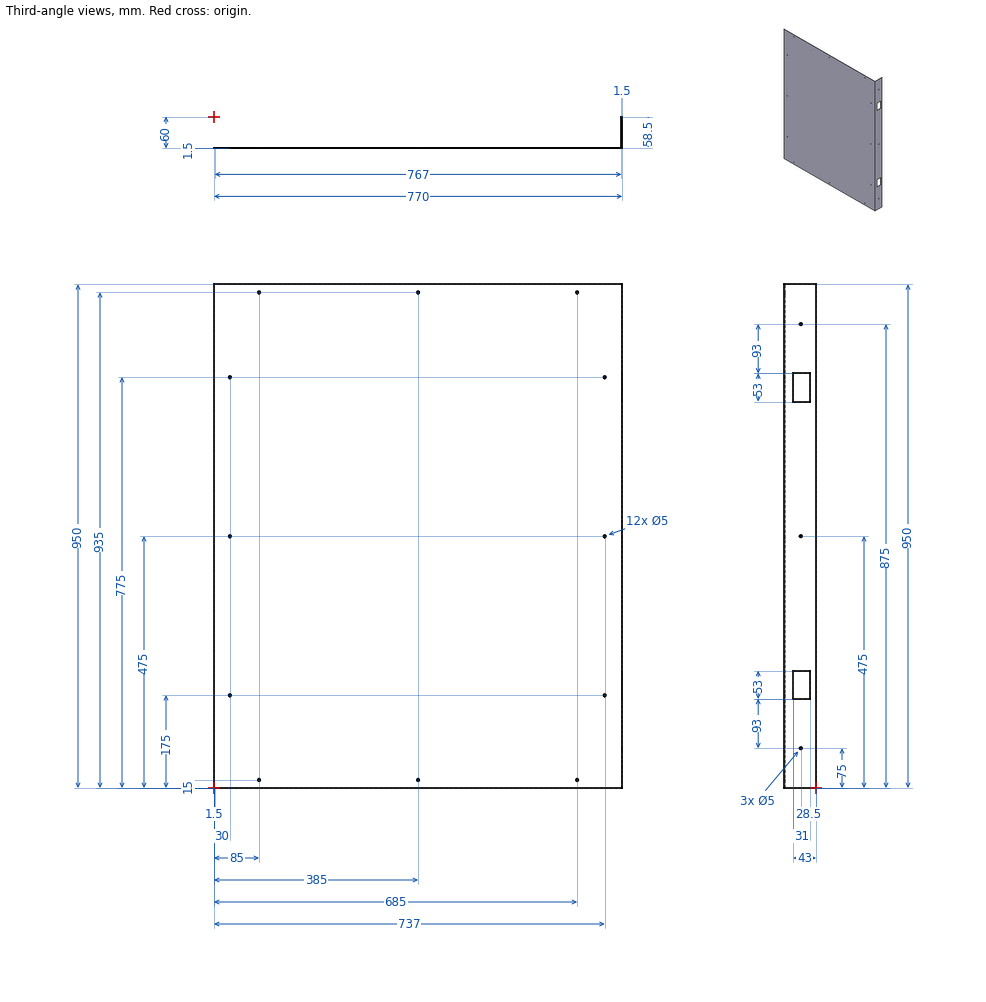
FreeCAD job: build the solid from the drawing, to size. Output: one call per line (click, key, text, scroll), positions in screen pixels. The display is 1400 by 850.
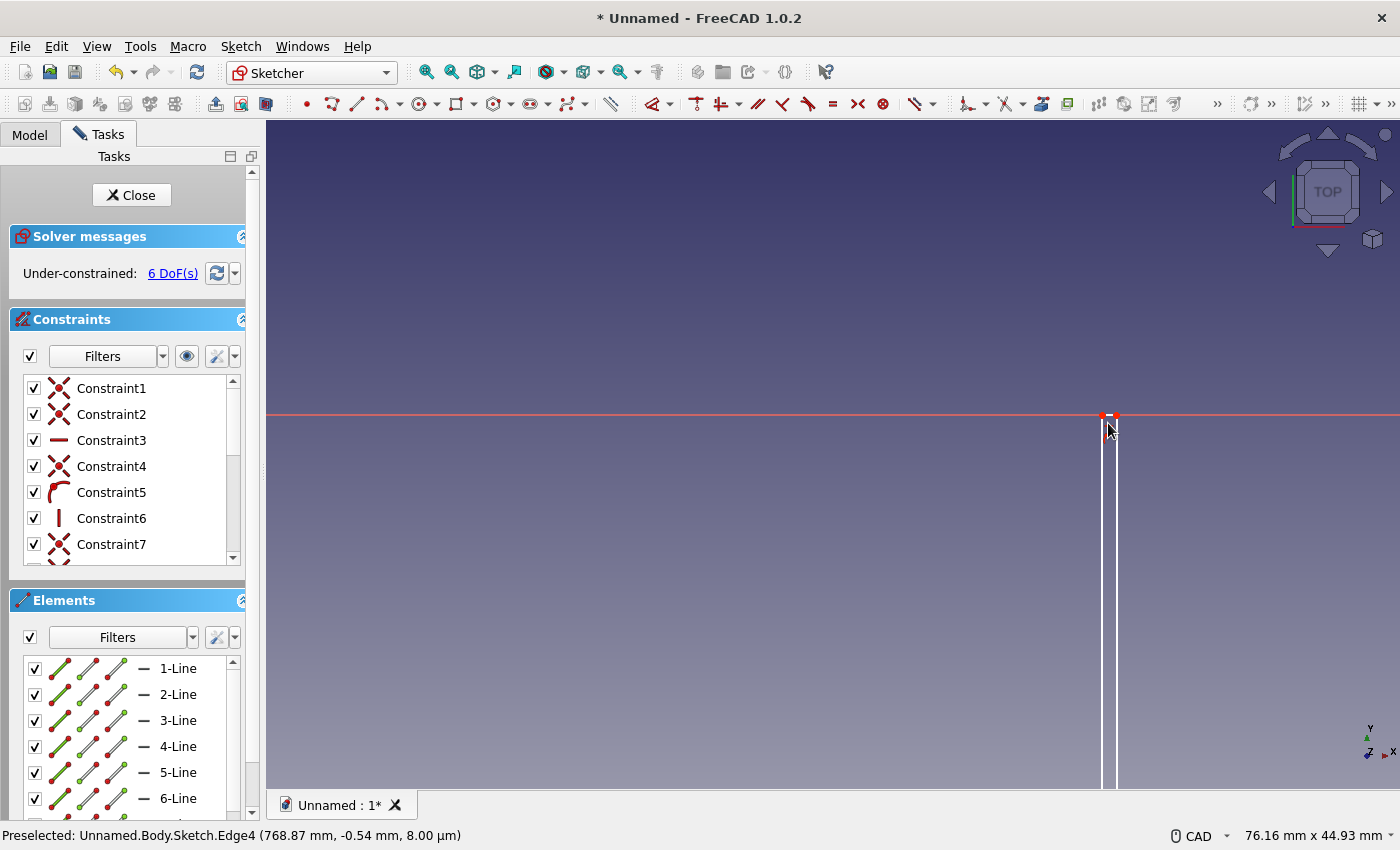
scroll(1112, 428, down, 14)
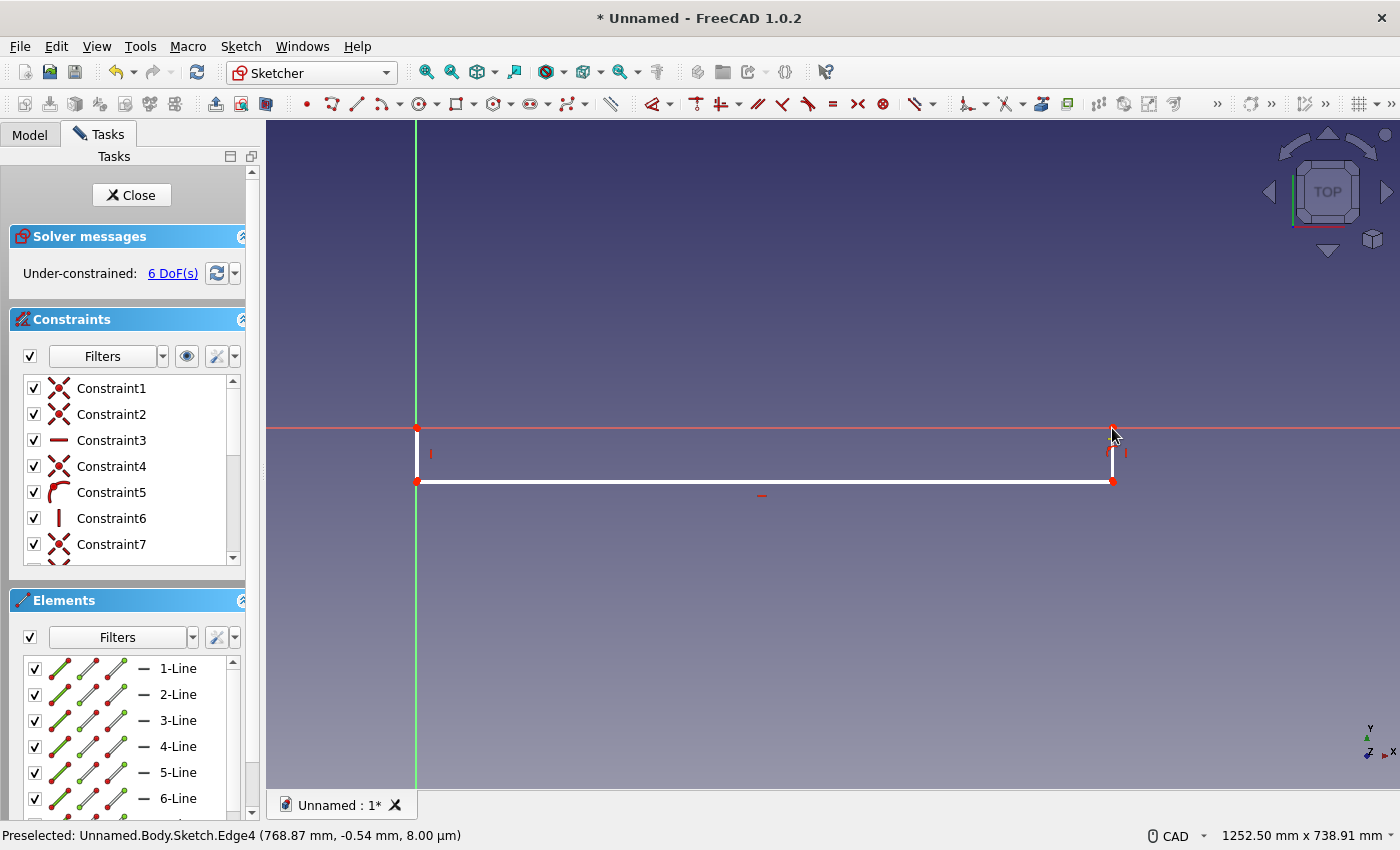
scroll(417, 428, up, 14)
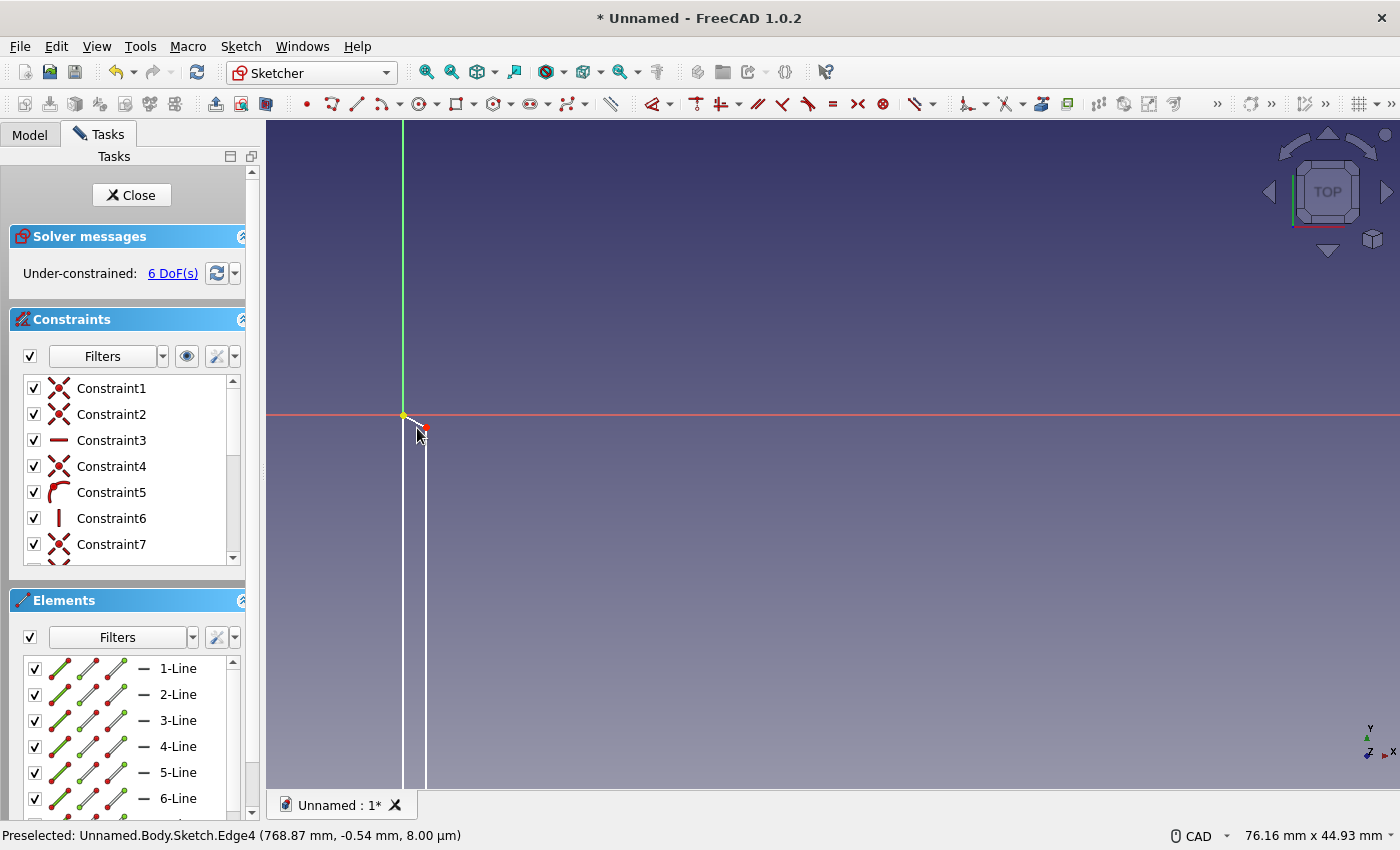
click(419, 424)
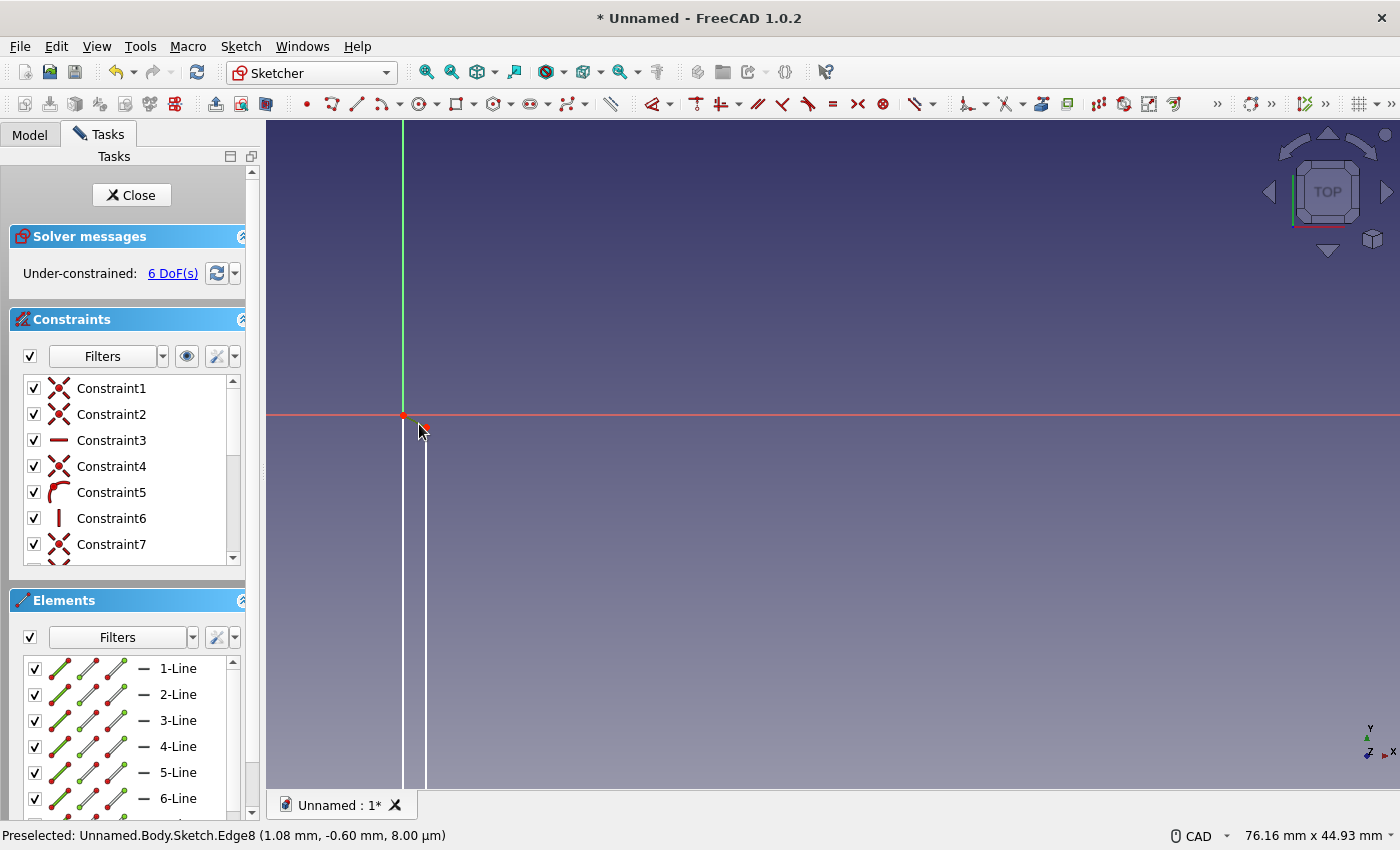
key(h)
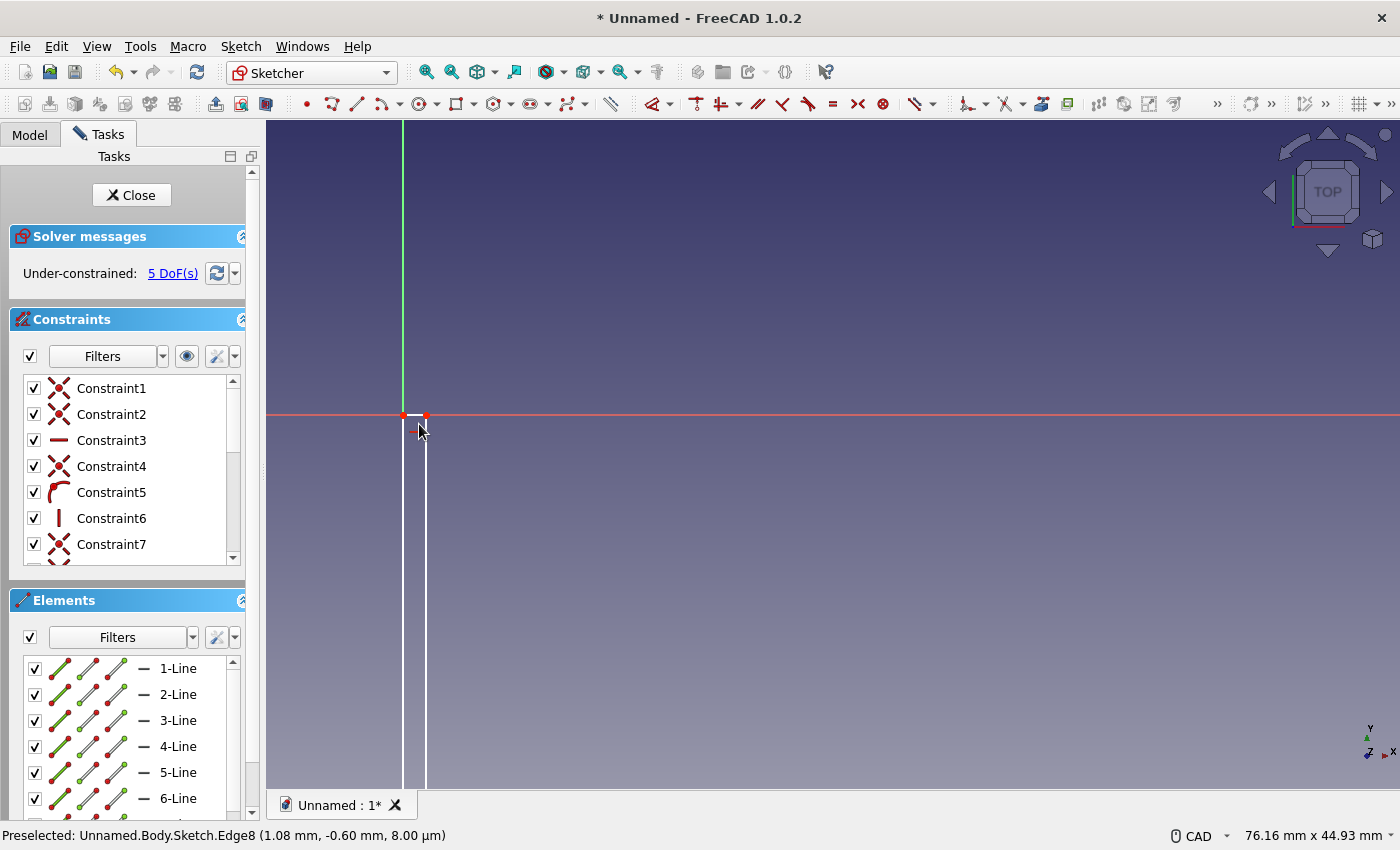
click(652, 104)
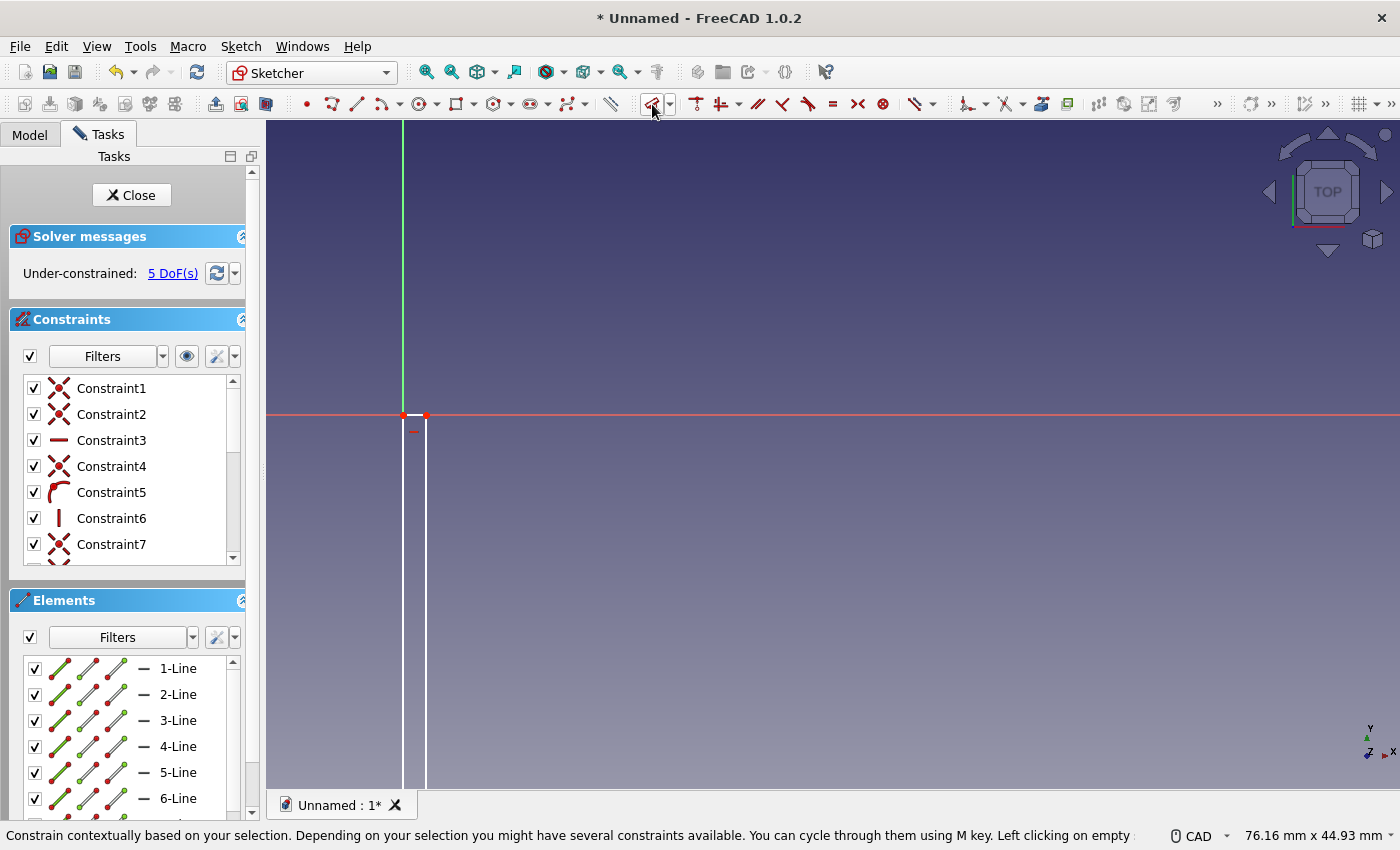
click(403, 688)
click(369, 588)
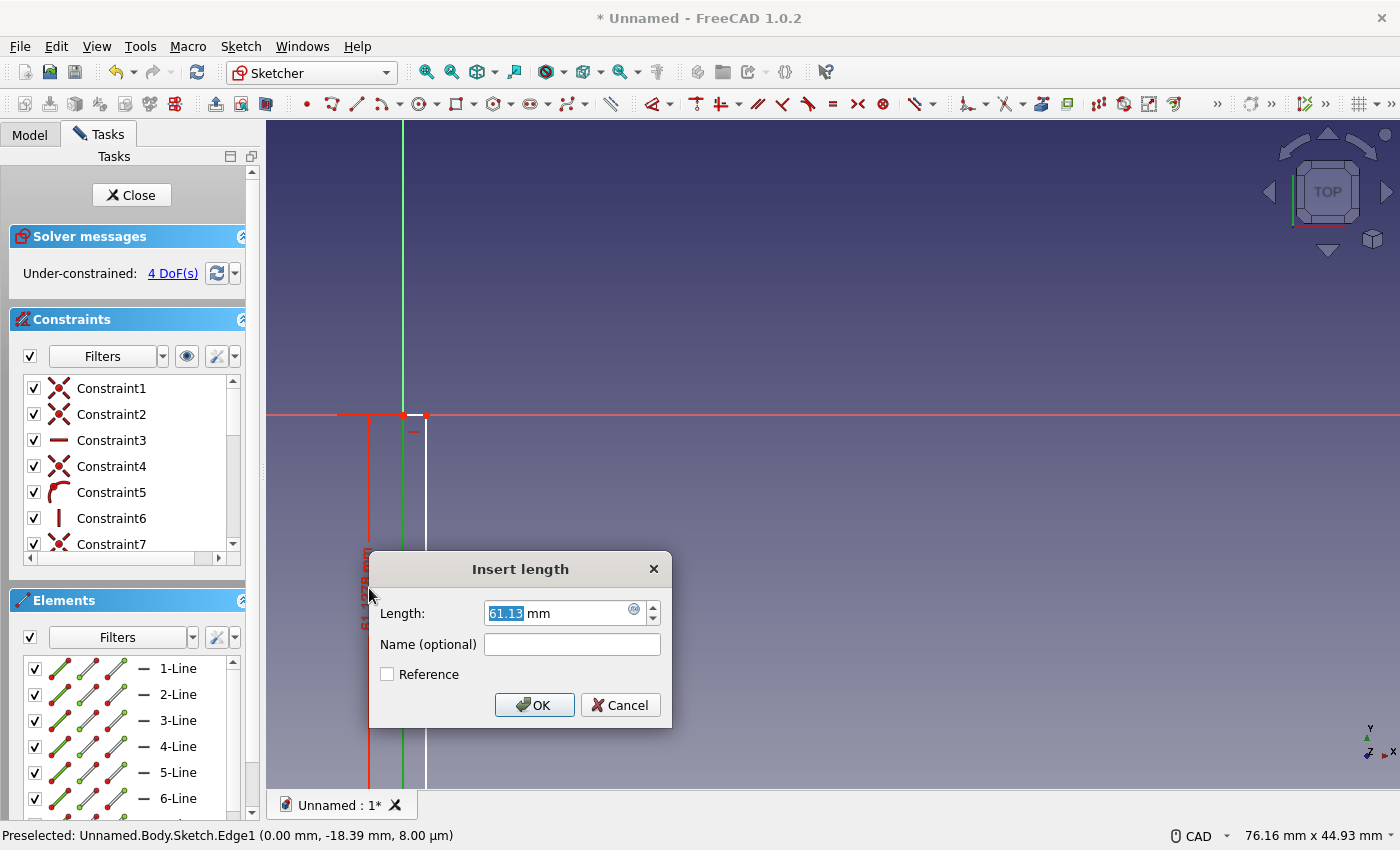
text(60)
key(Return)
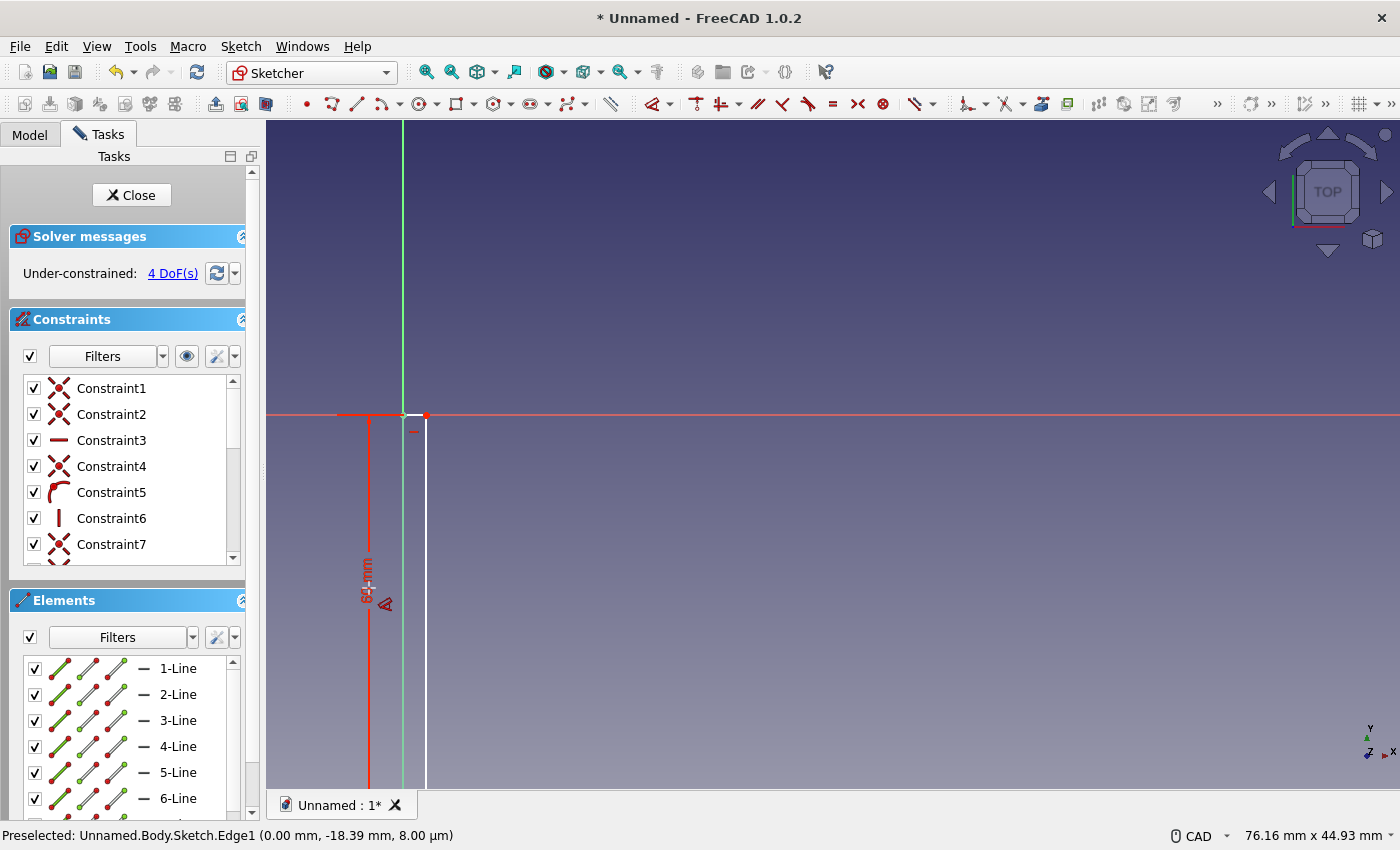
scroll(417, 428, down, 14)